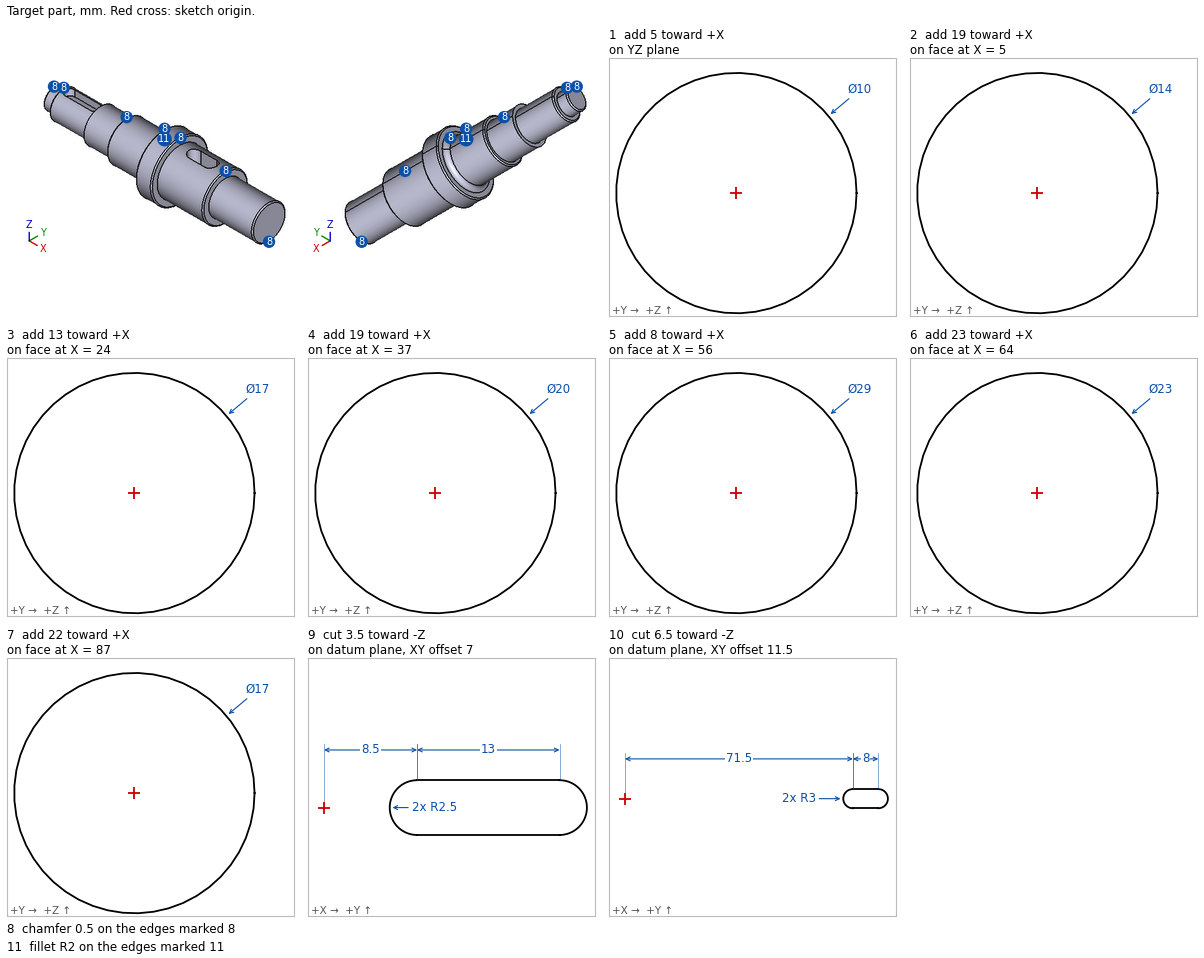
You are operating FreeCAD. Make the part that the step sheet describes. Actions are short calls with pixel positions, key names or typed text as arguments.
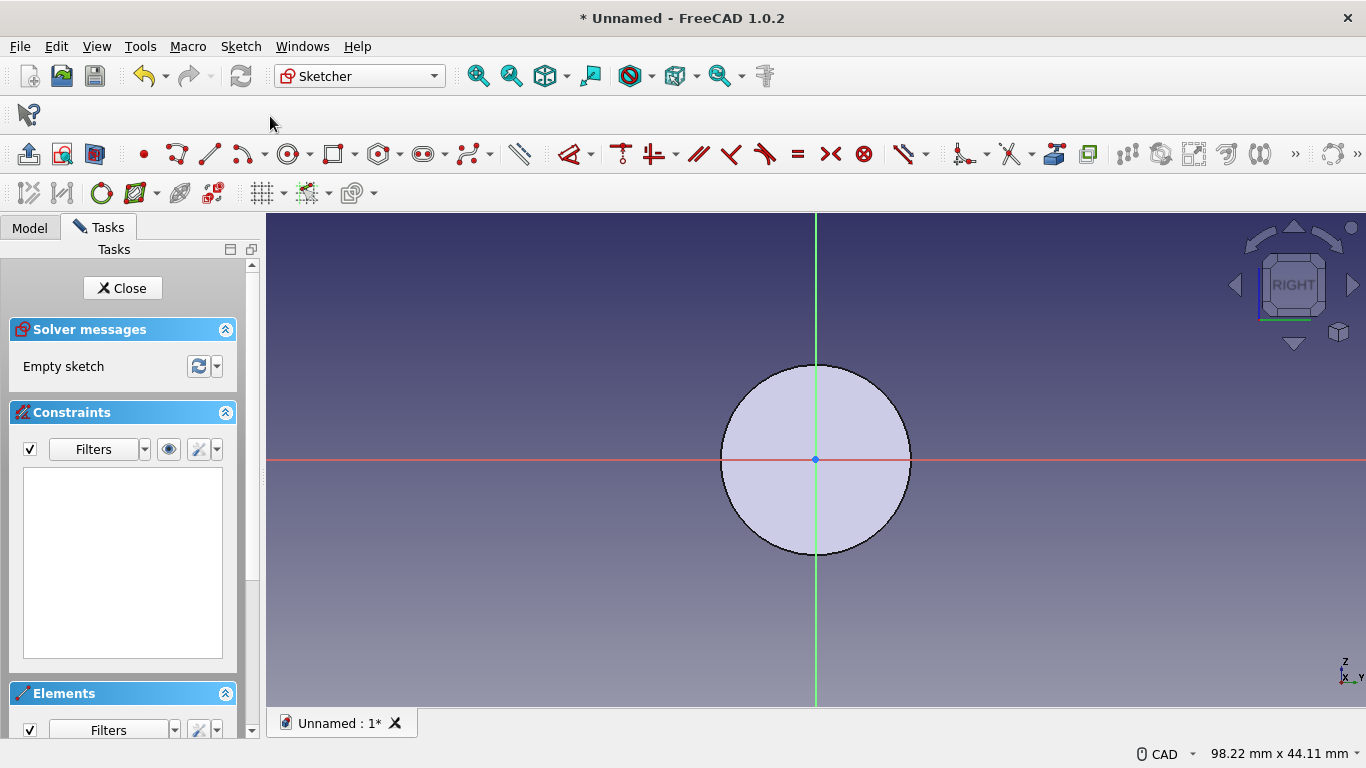
scroll(955, 460, up, 2)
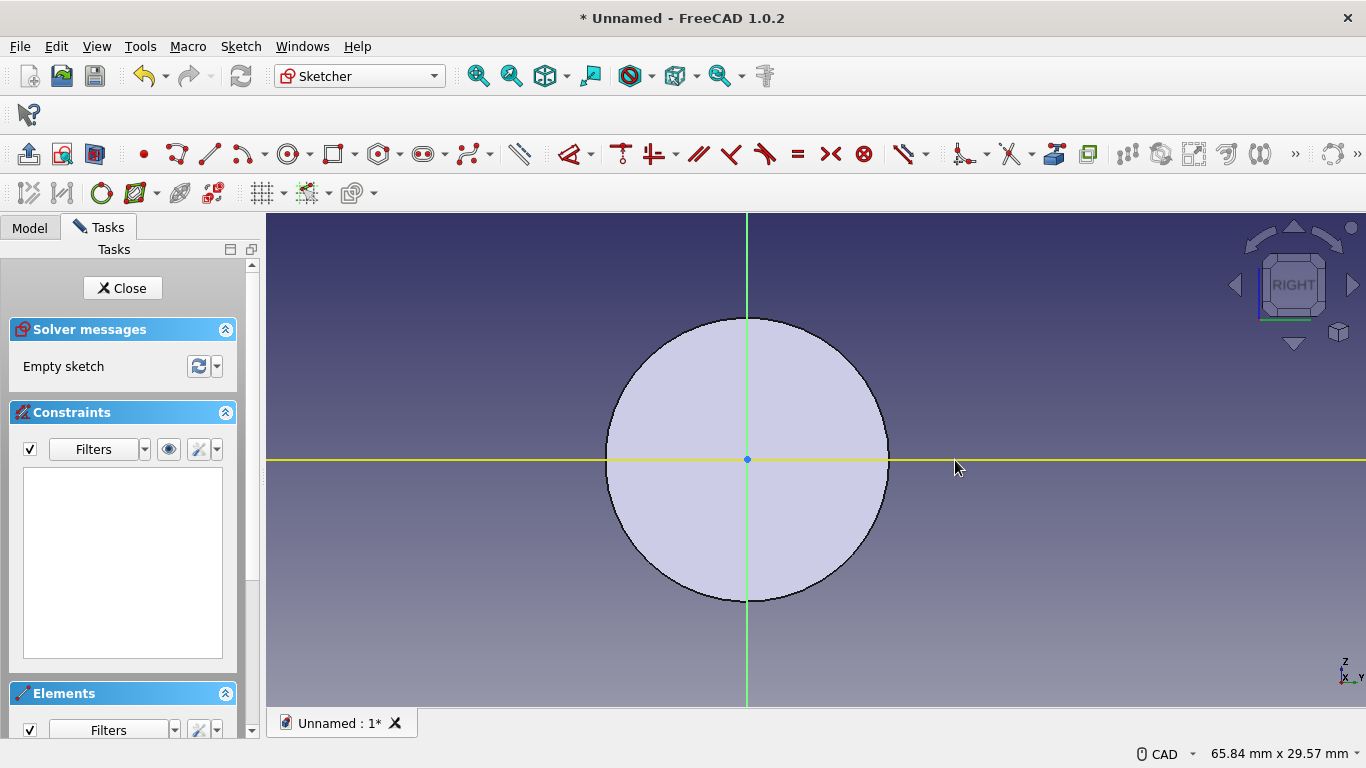
click(288, 154)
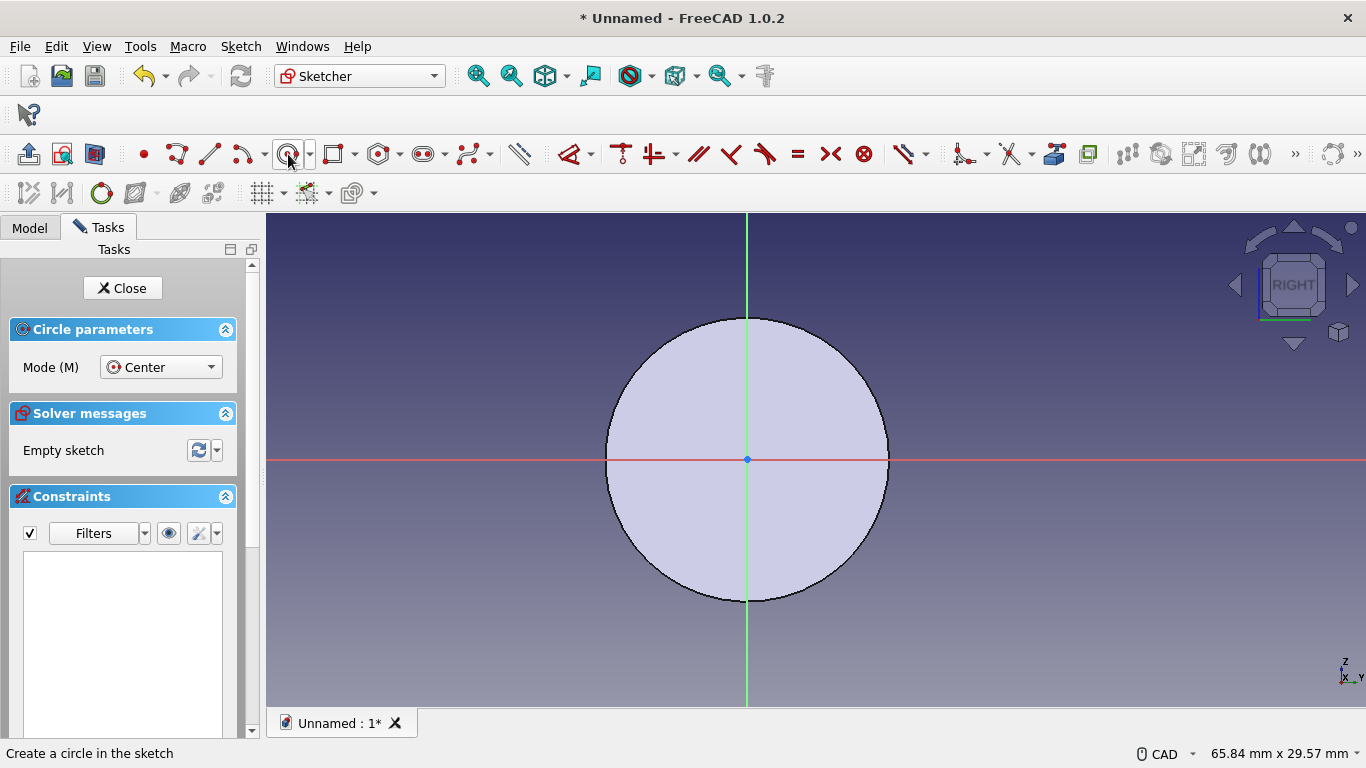
click(747, 460)
move(865, 342)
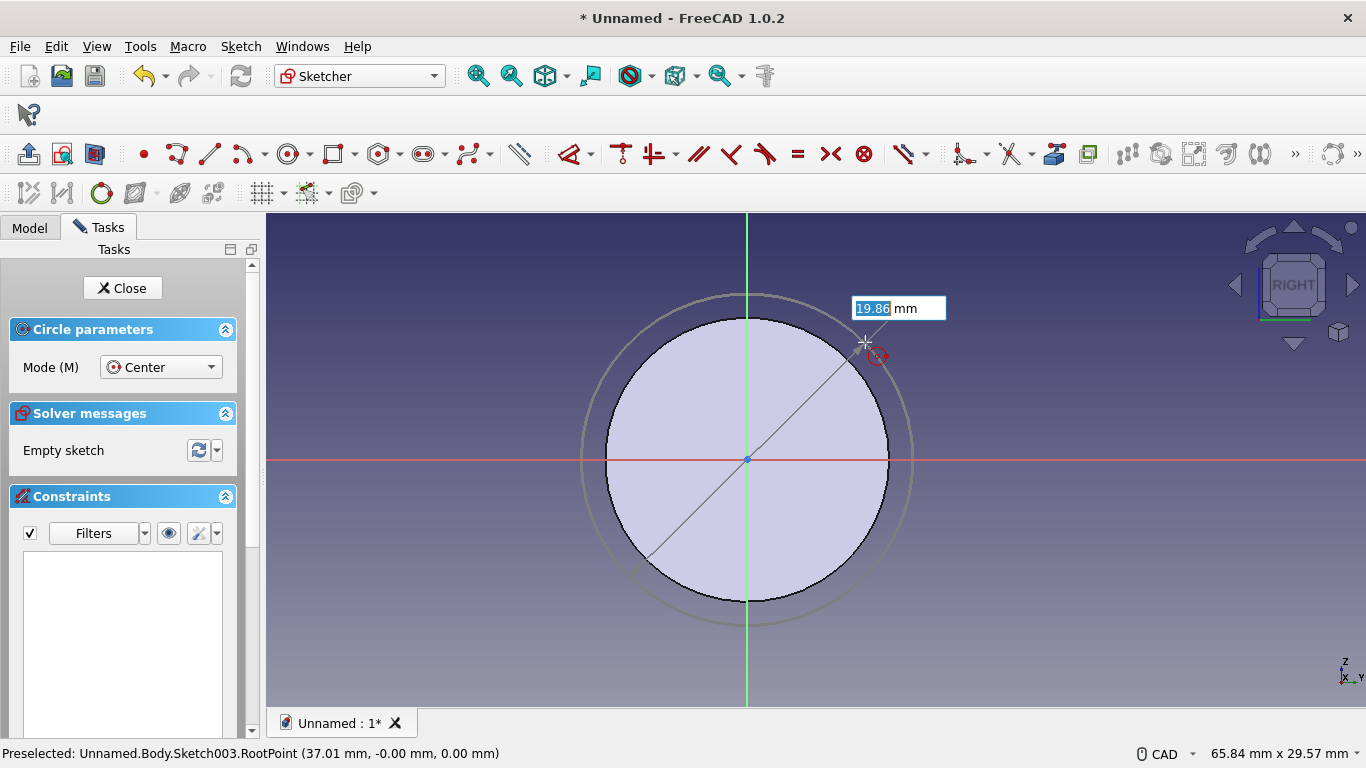
text(20)
key(Return)
key(Escape)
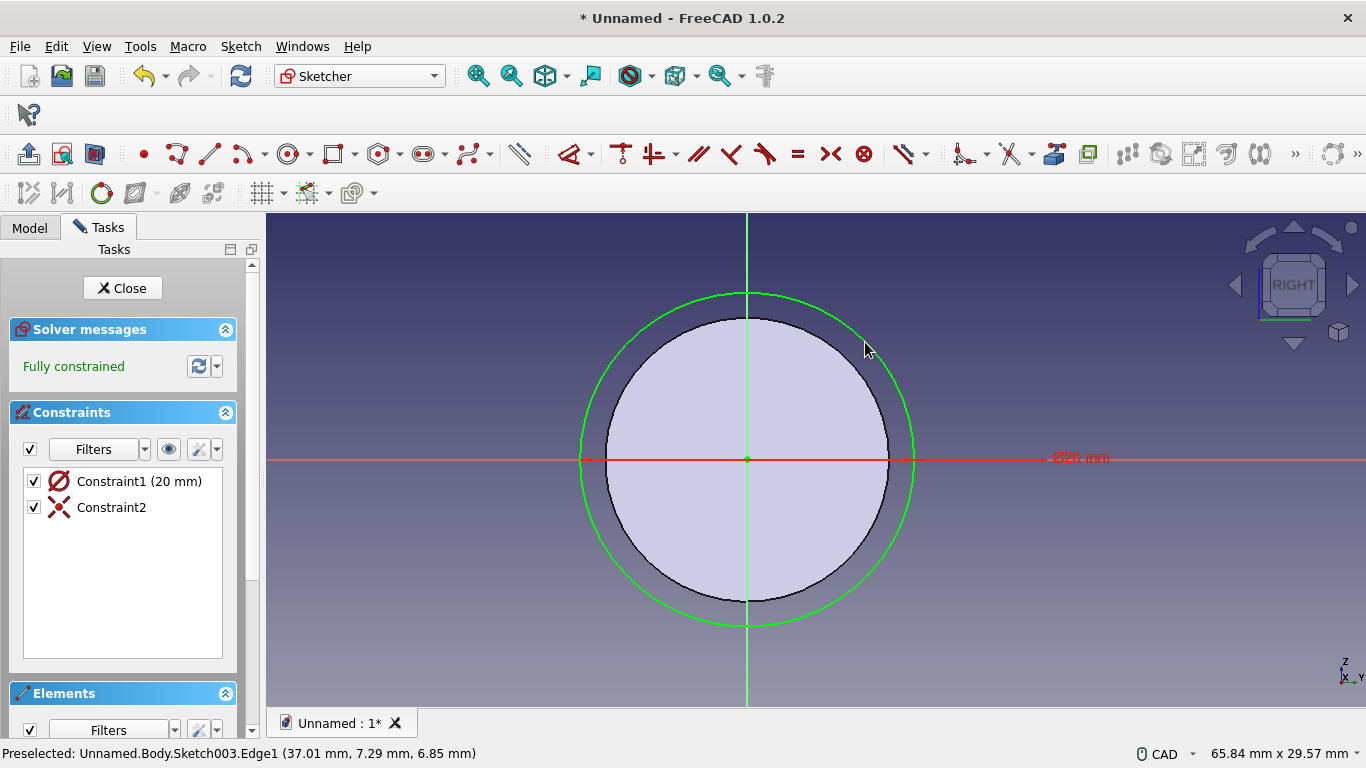
click(123, 288)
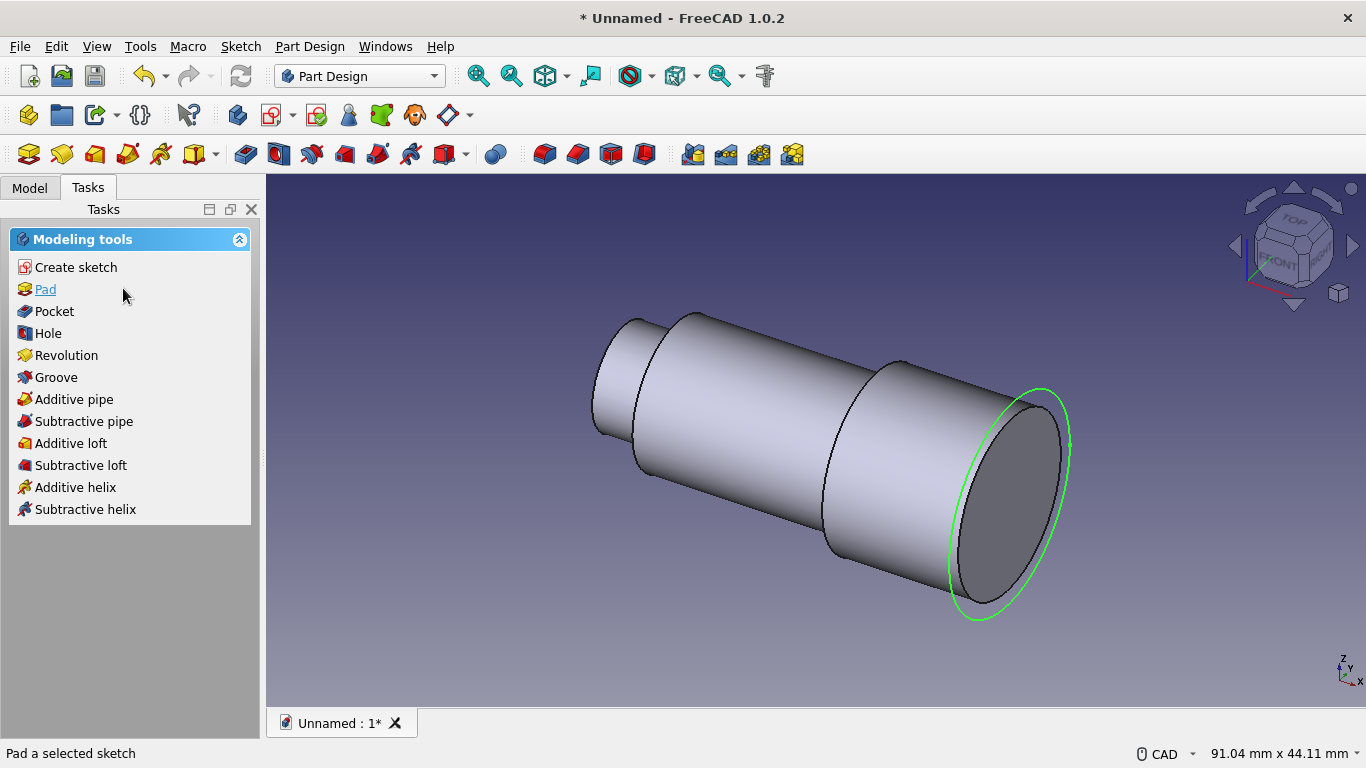
click(29, 154)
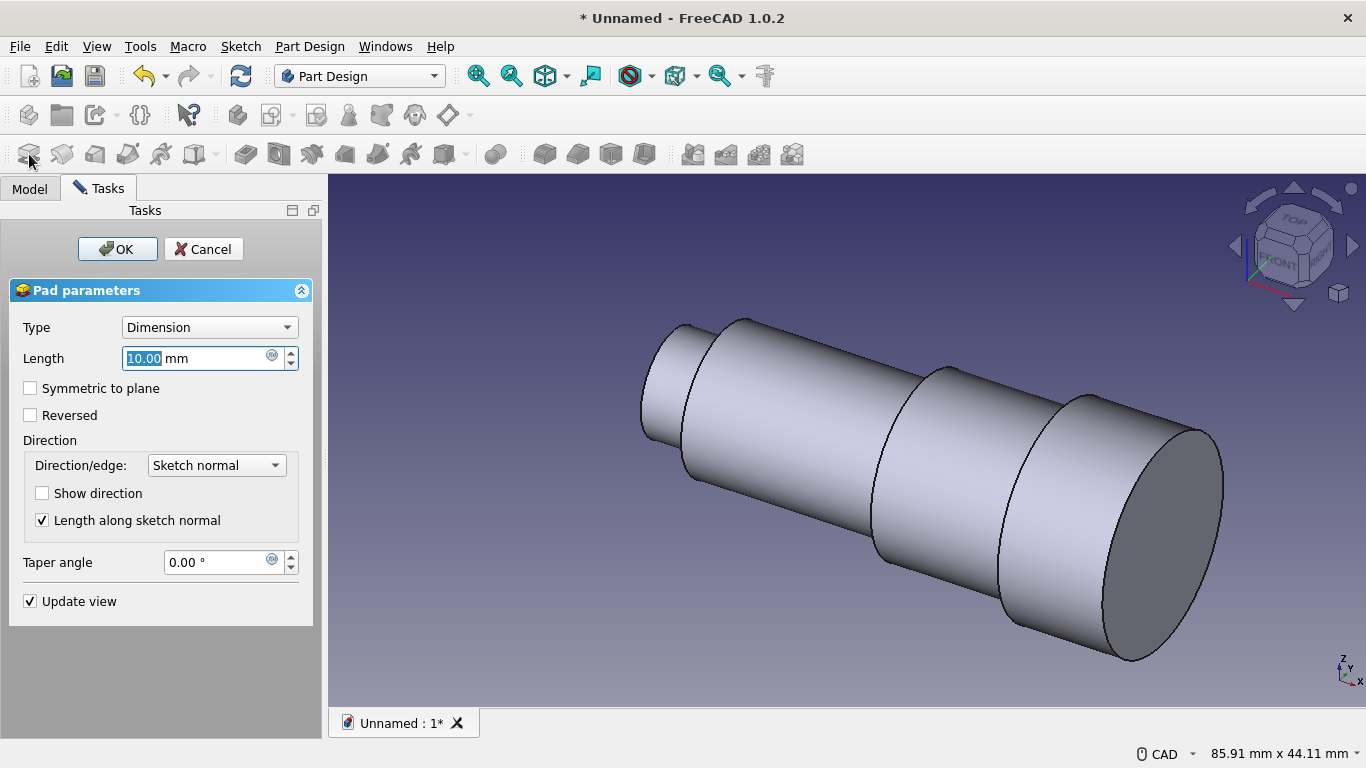
text(19)
key(Tab)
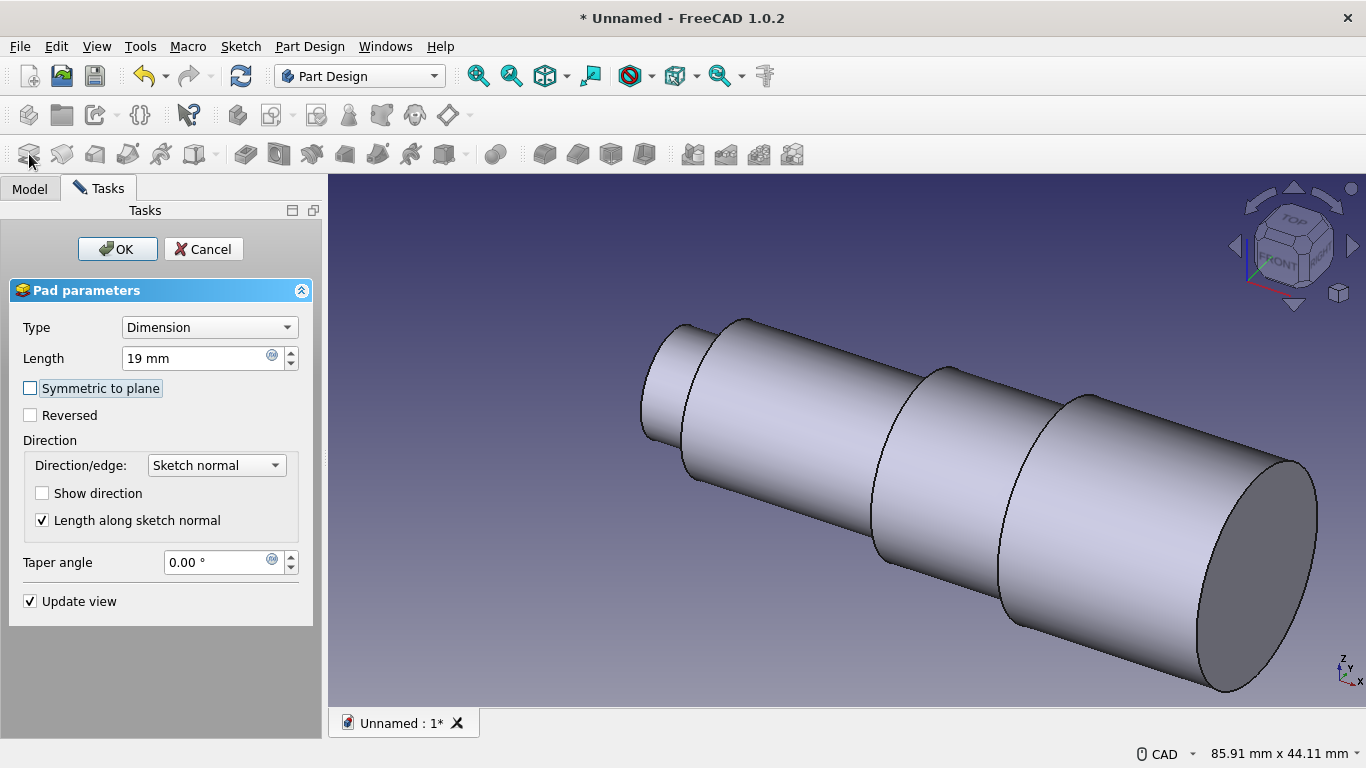
click(118, 249)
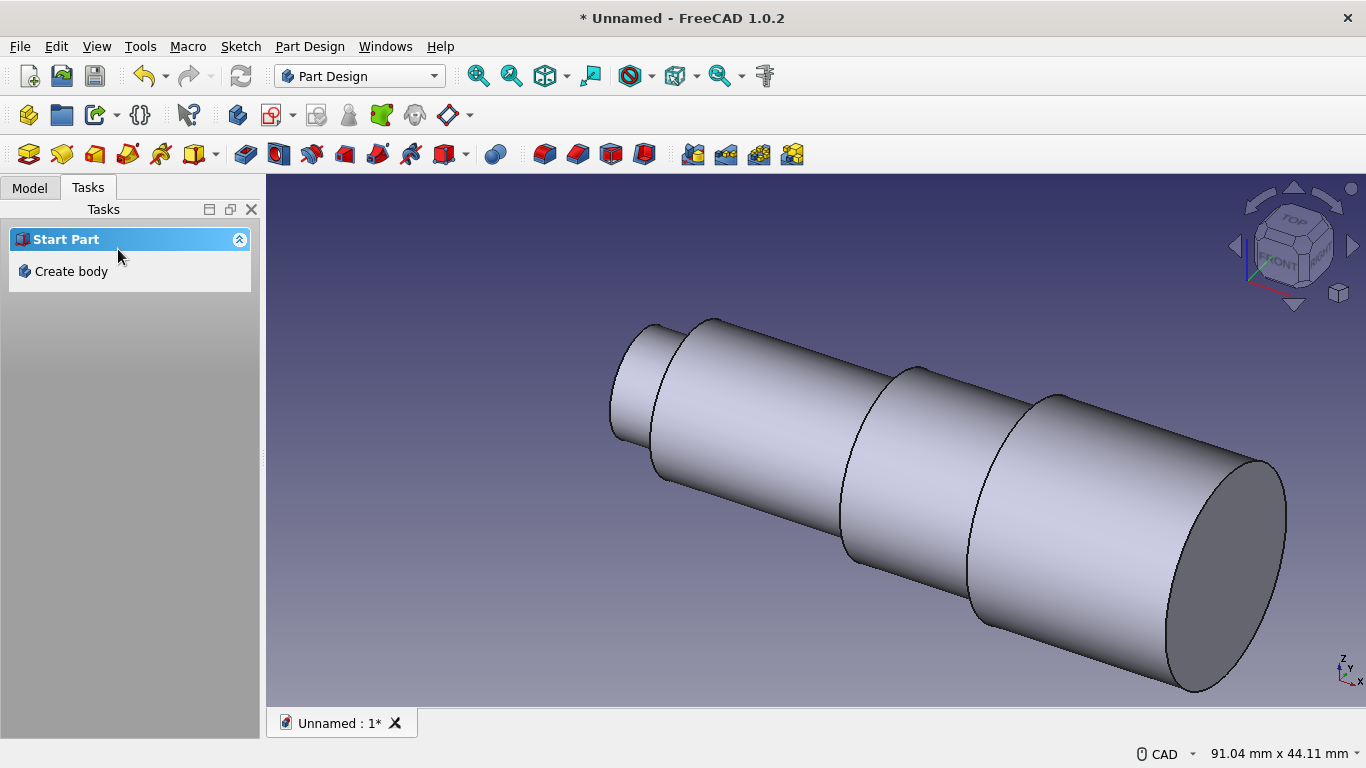
click(479, 76)